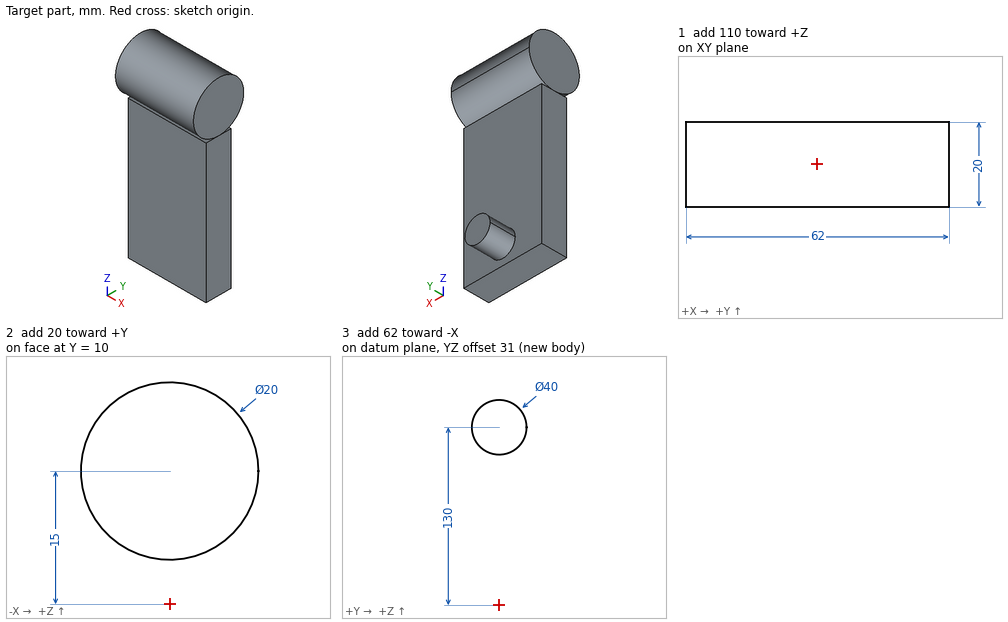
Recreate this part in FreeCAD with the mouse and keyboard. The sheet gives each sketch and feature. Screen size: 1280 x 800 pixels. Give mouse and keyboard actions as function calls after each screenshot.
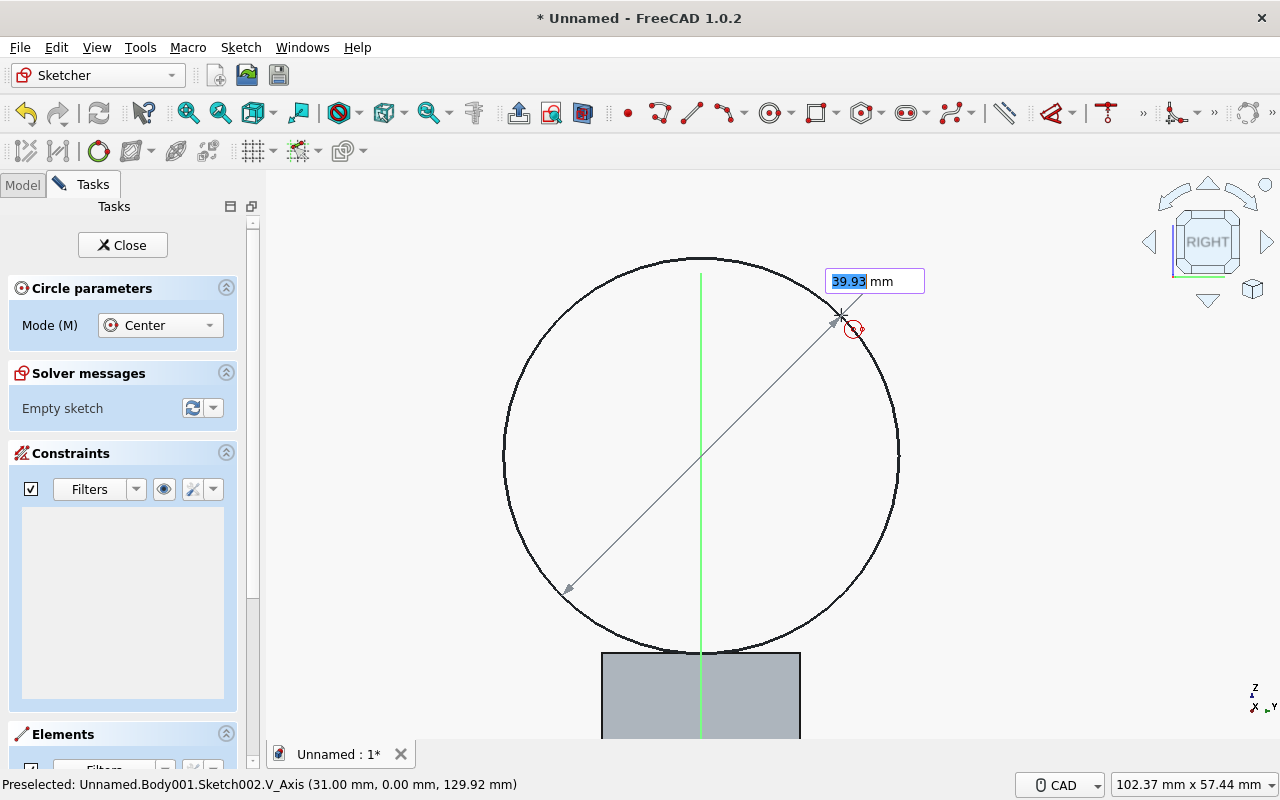
text(40)
key(Return)
key(Escape)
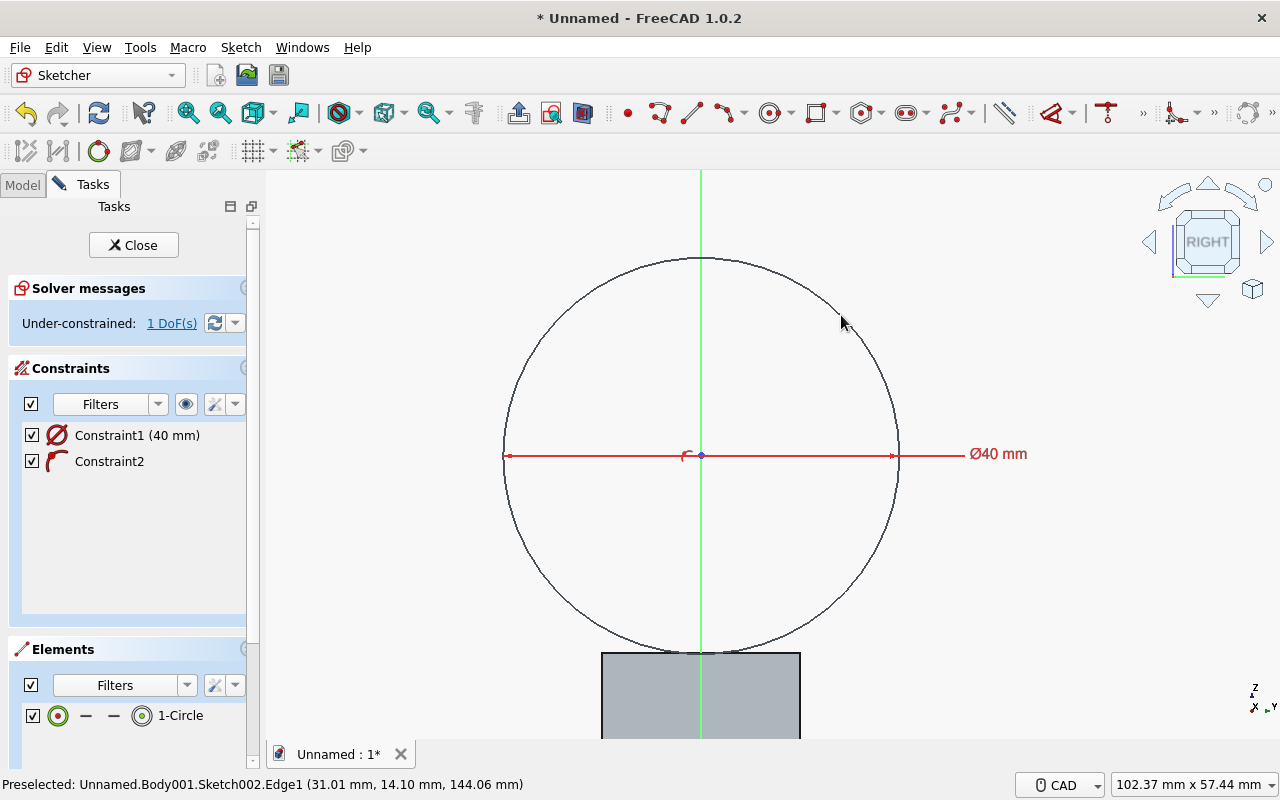
key(d)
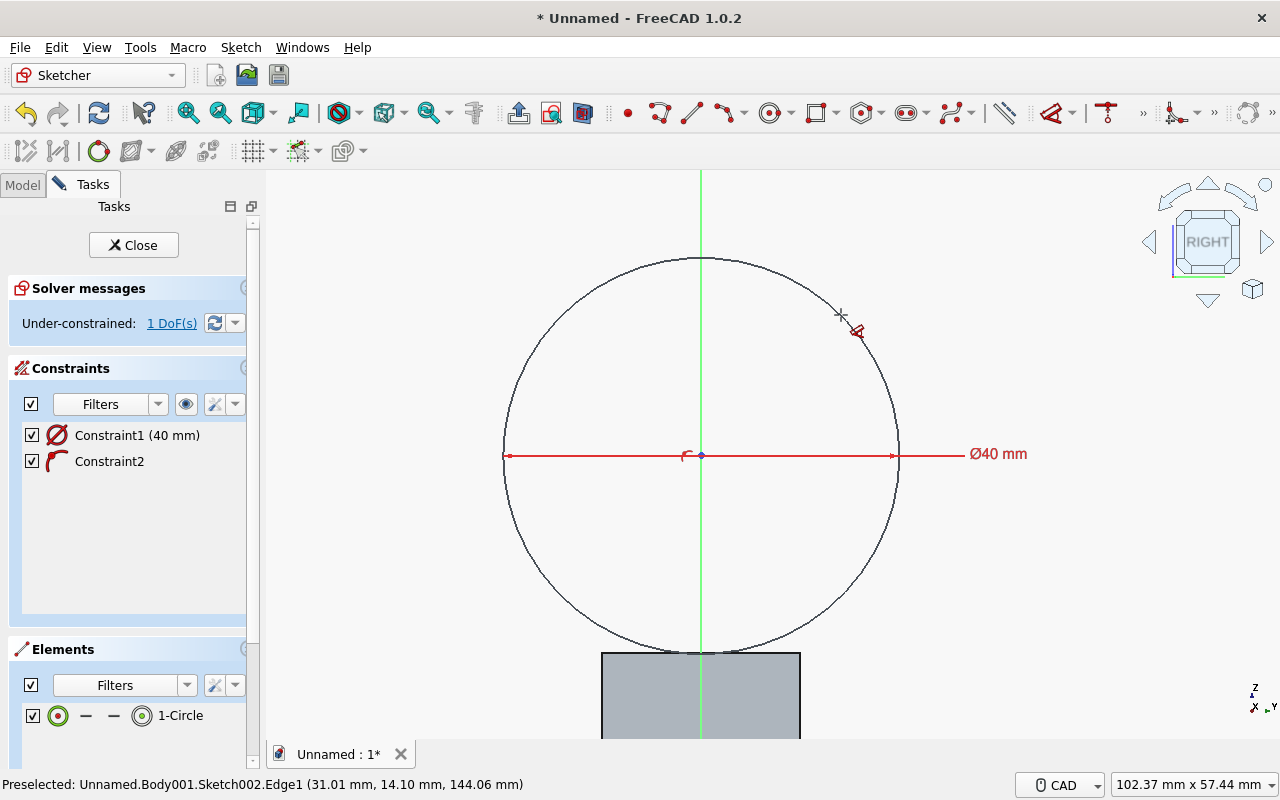
click(701, 456)
click(735, 583)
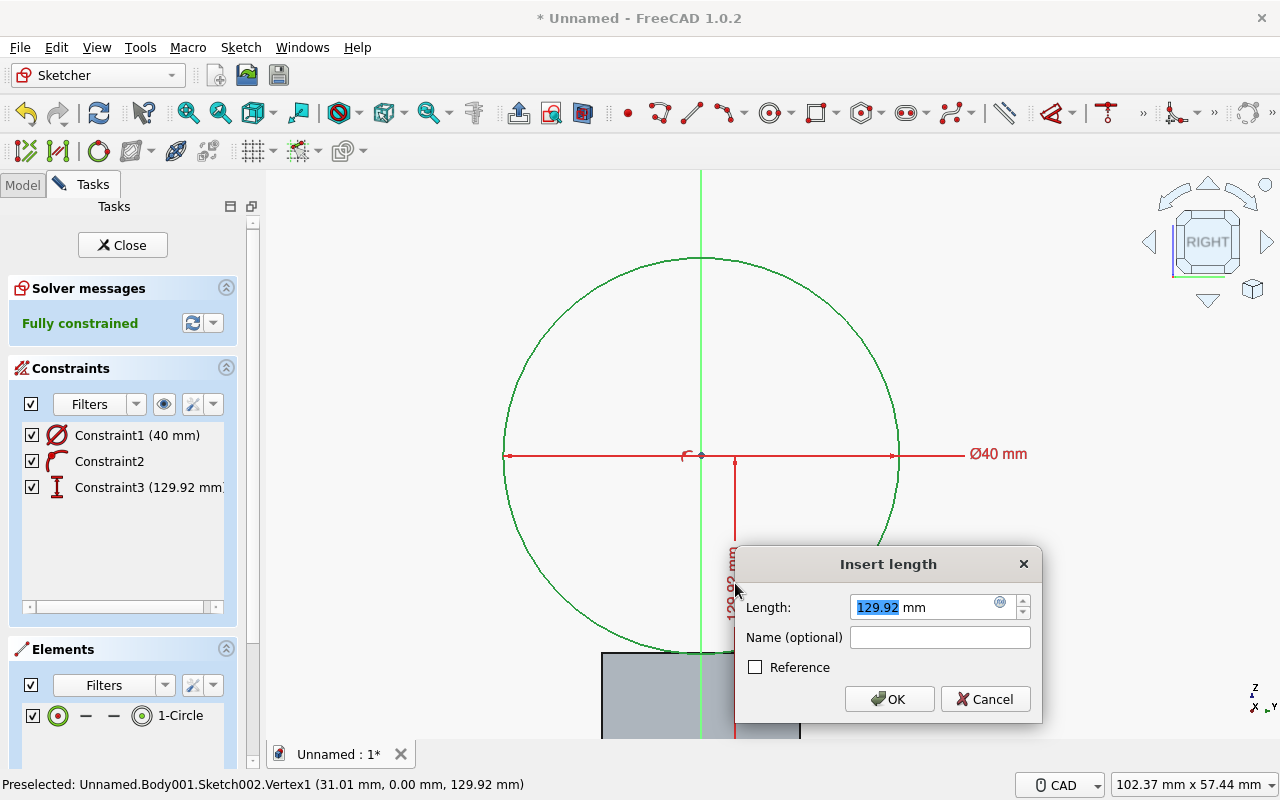
text(130)
key(Return)
key(Escape)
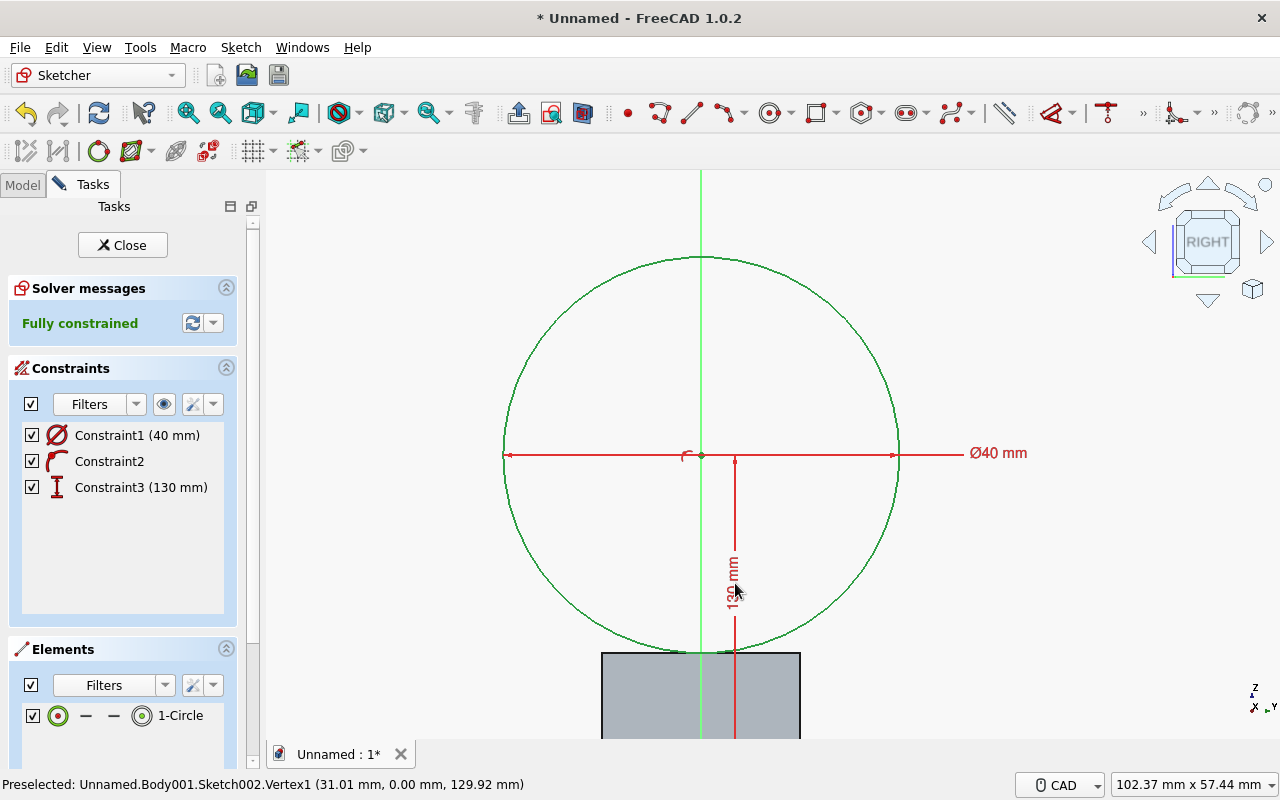
click(123, 245)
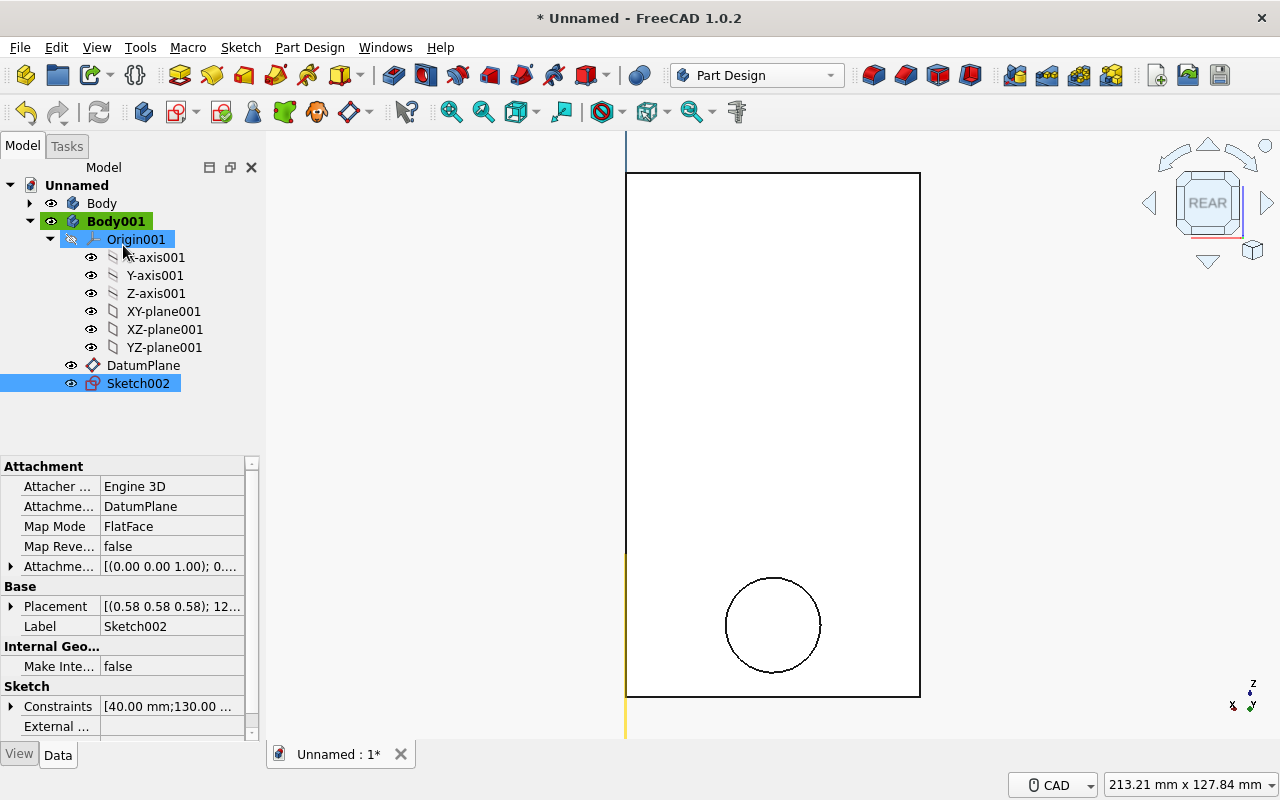
click(180, 76)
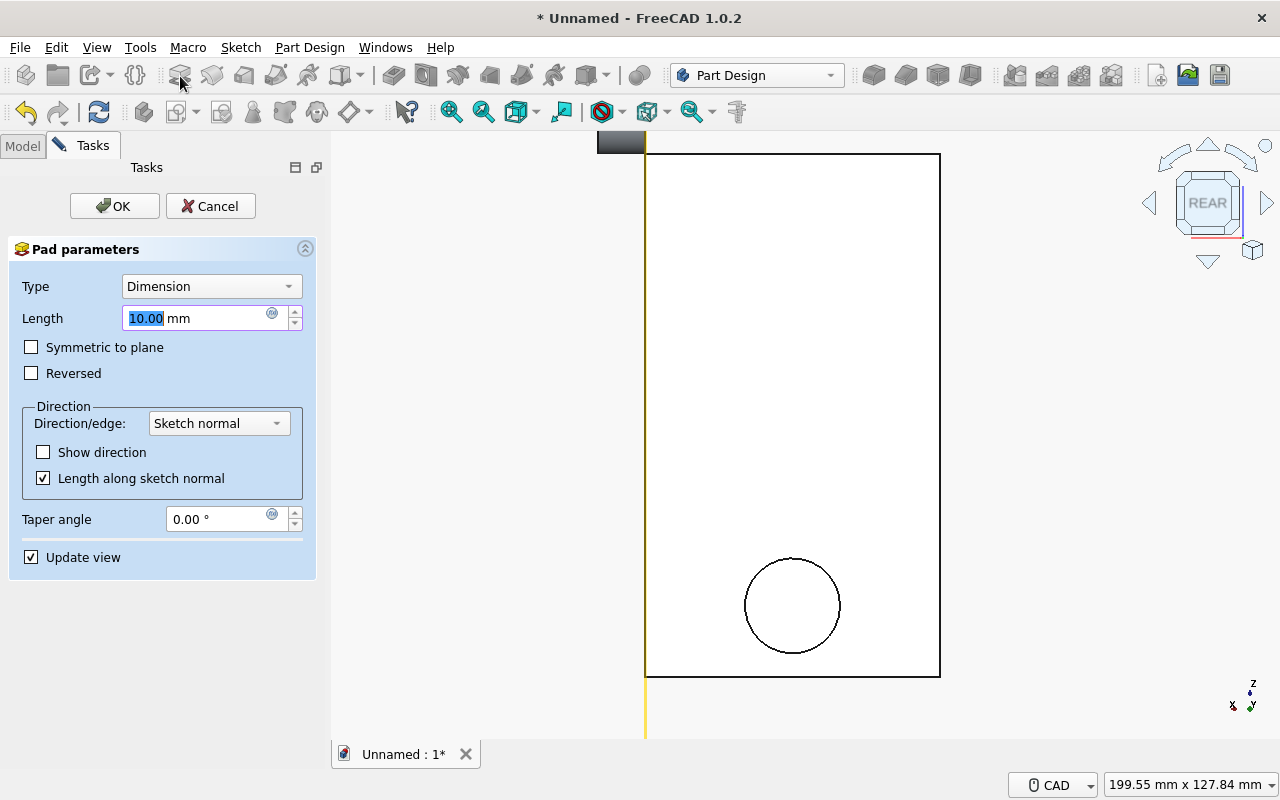
text(62)
key(Tab)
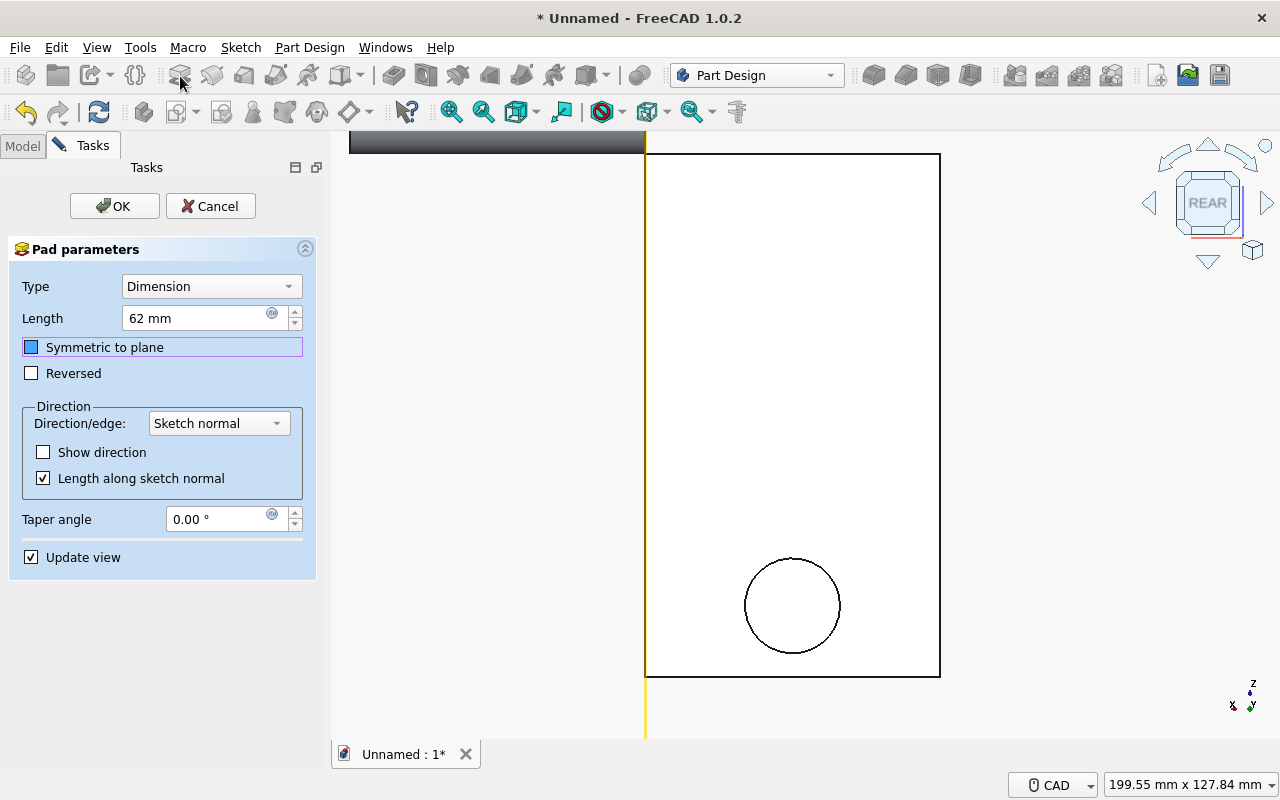
click(30, 373)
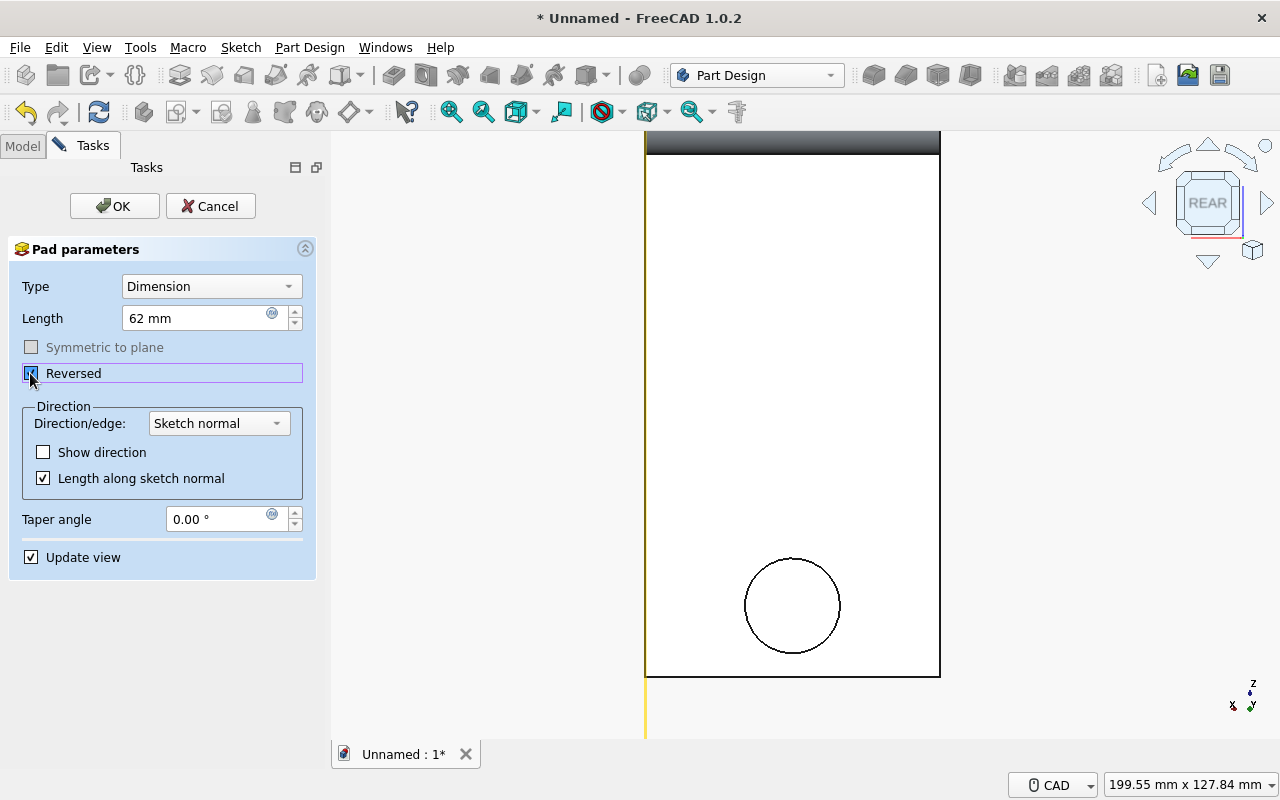
click(115, 206)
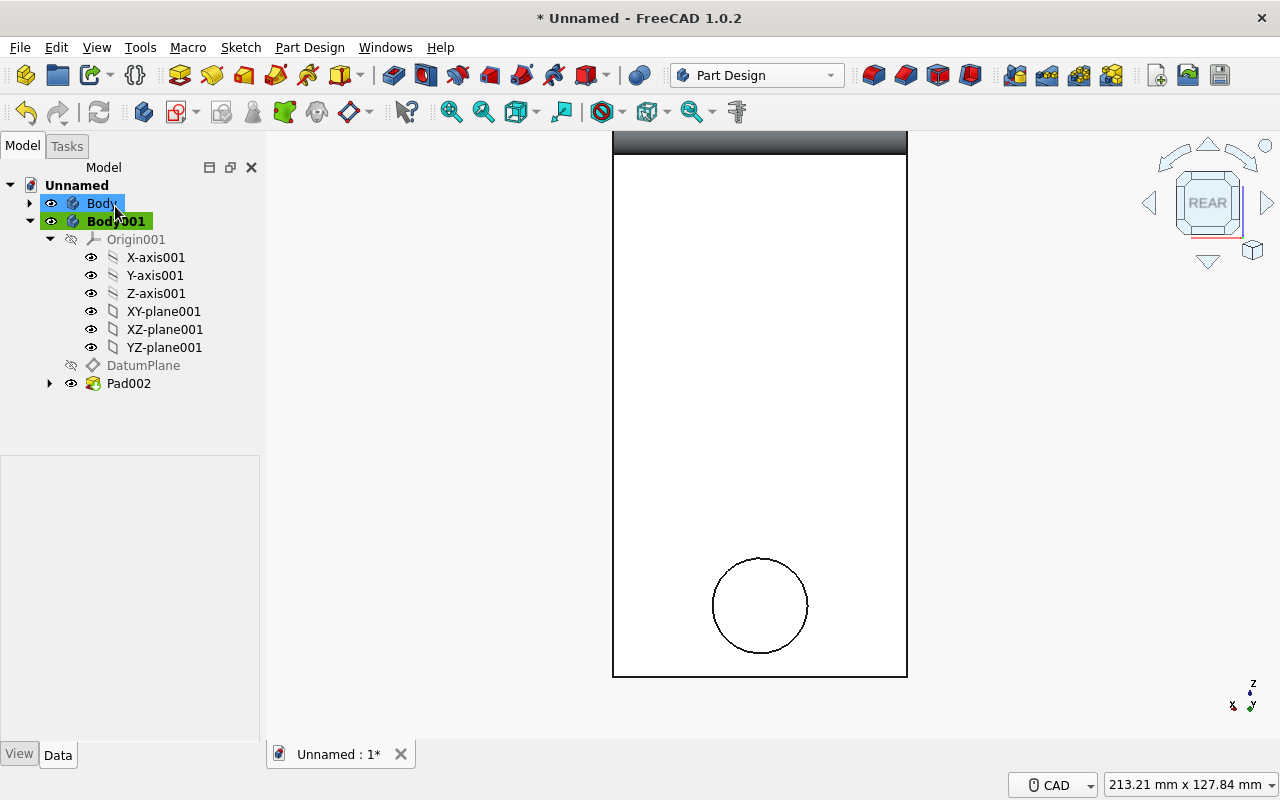
key(0)